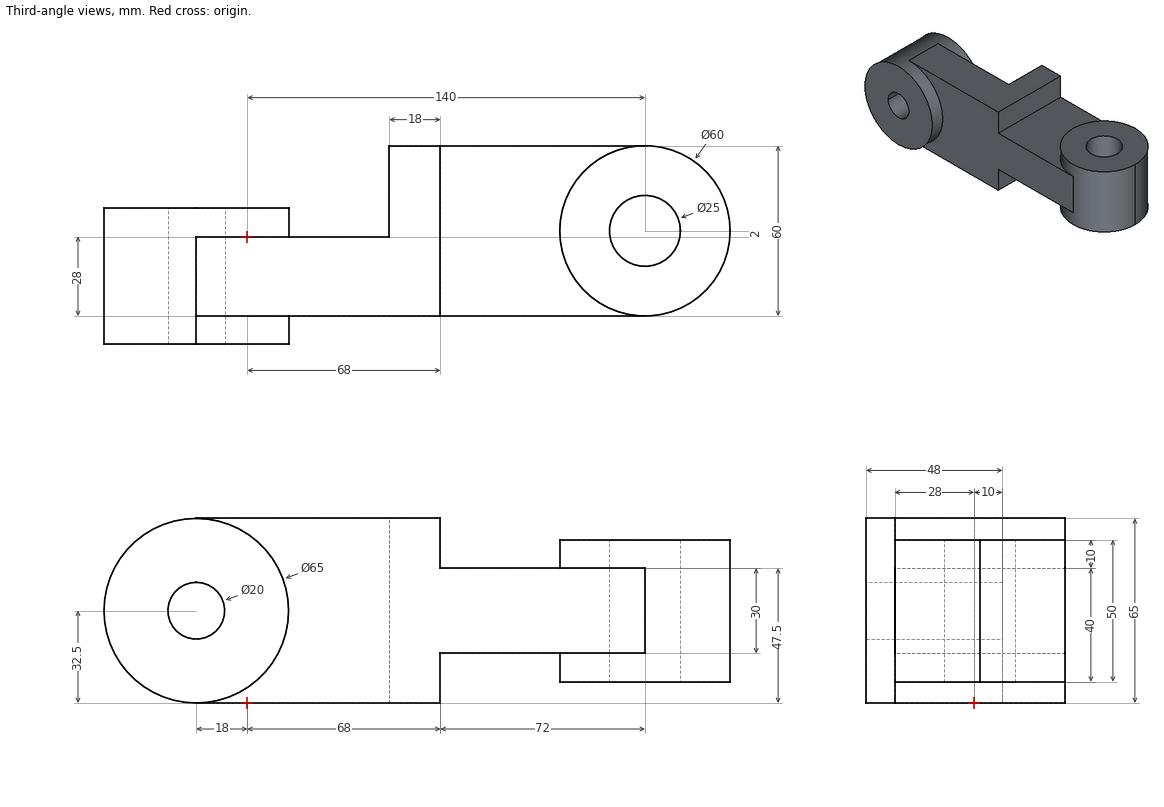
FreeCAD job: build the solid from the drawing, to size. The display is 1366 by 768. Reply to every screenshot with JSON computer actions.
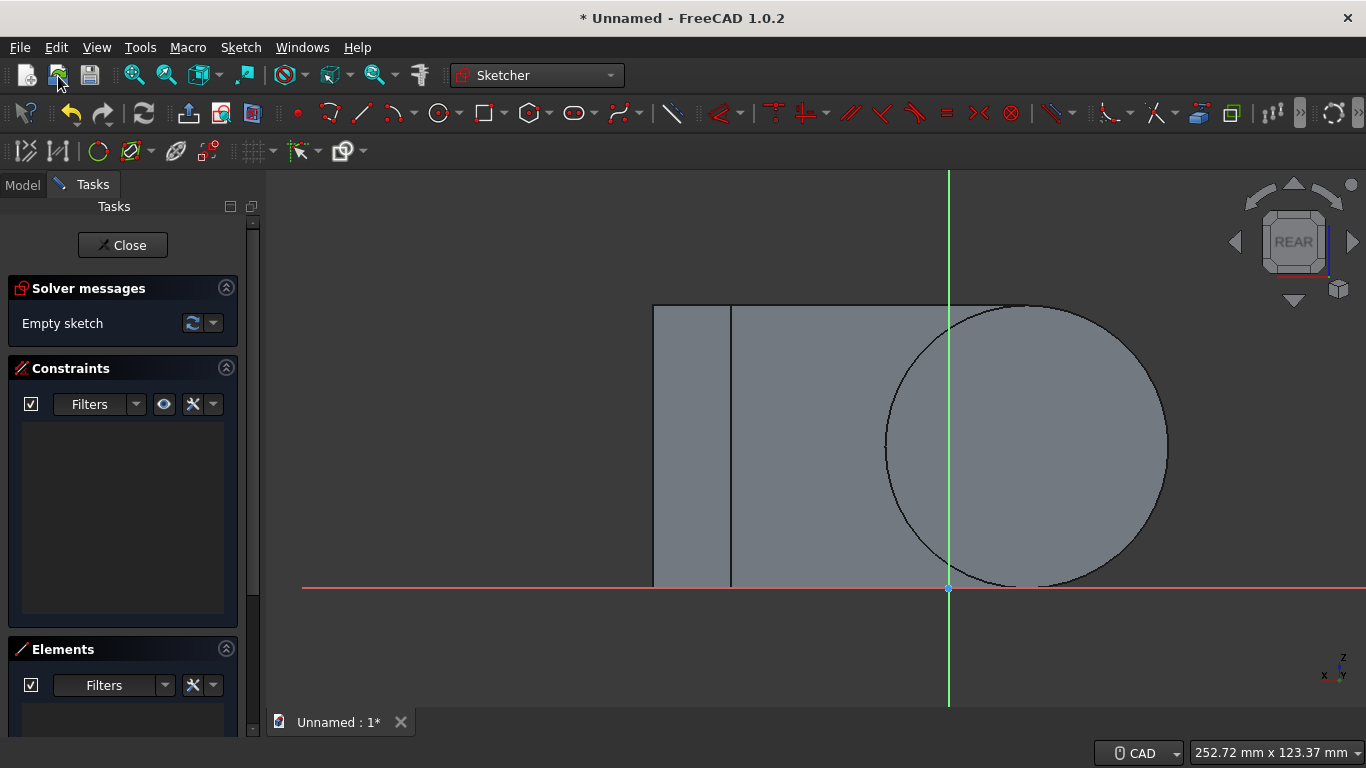
{"action": "scroll", "coordinate": [1201, 565], "scroll_direction": "up", "scroll_amount": 3}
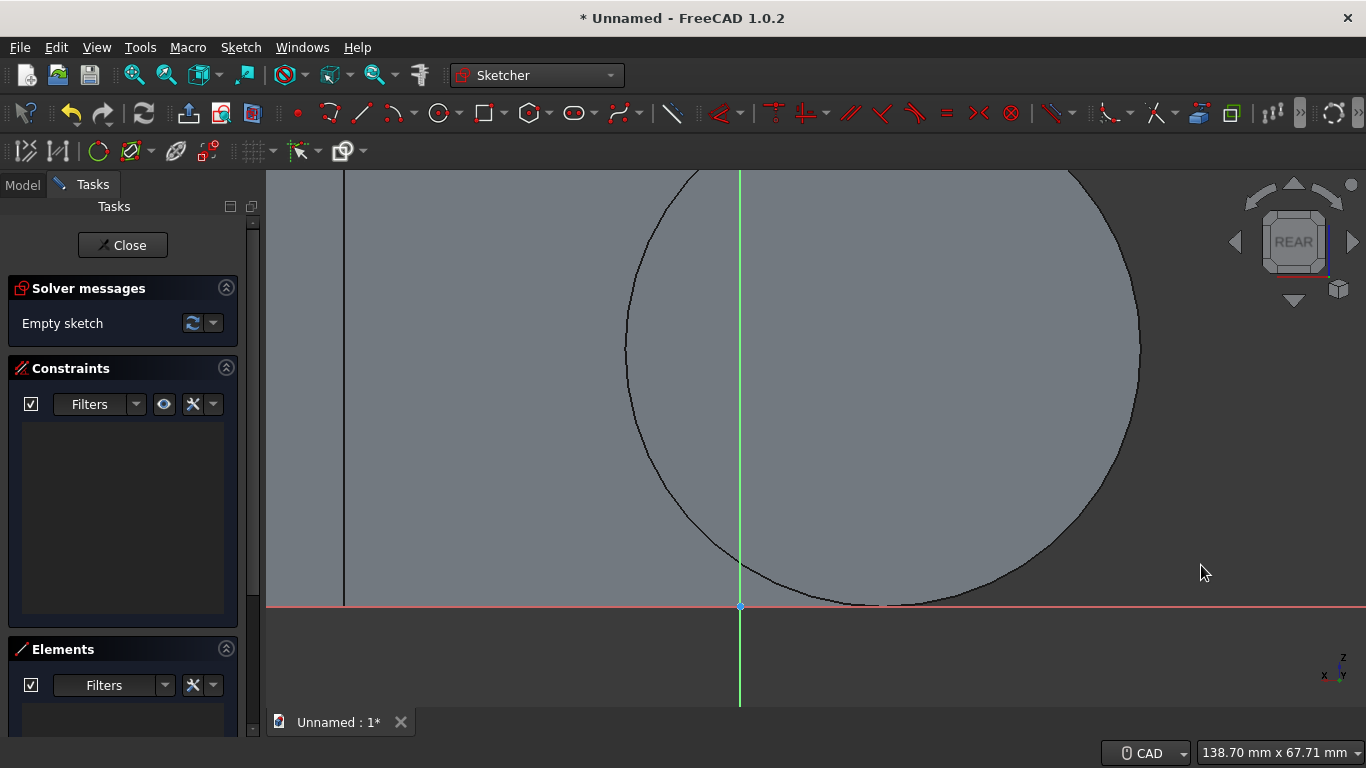
{"action": "key", "text": "g c"}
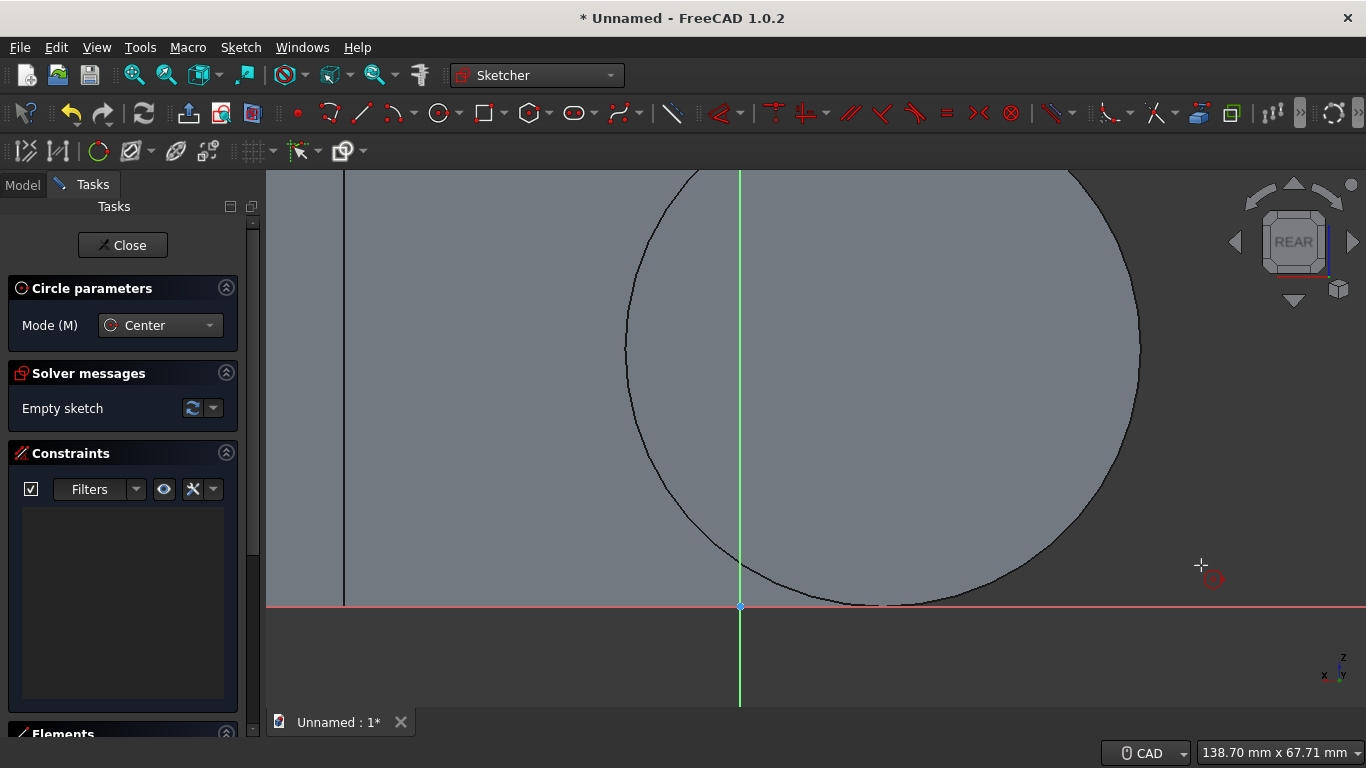
{"action": "left_click", "coordinate": [883, 349]}
{"action": "left_click", "coordinate": [939, 293]}
{"action": "key", "text": "Escape"}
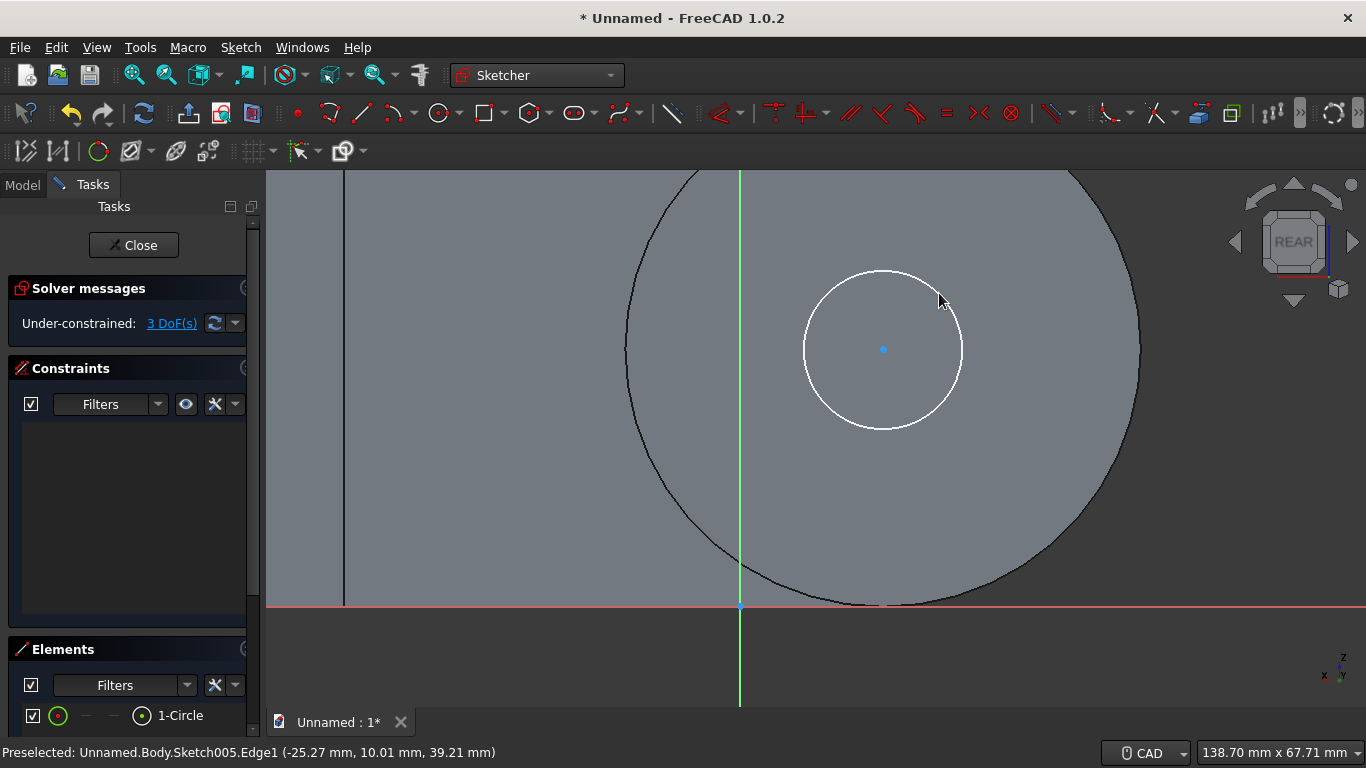
{"action": "key", "text": "d"}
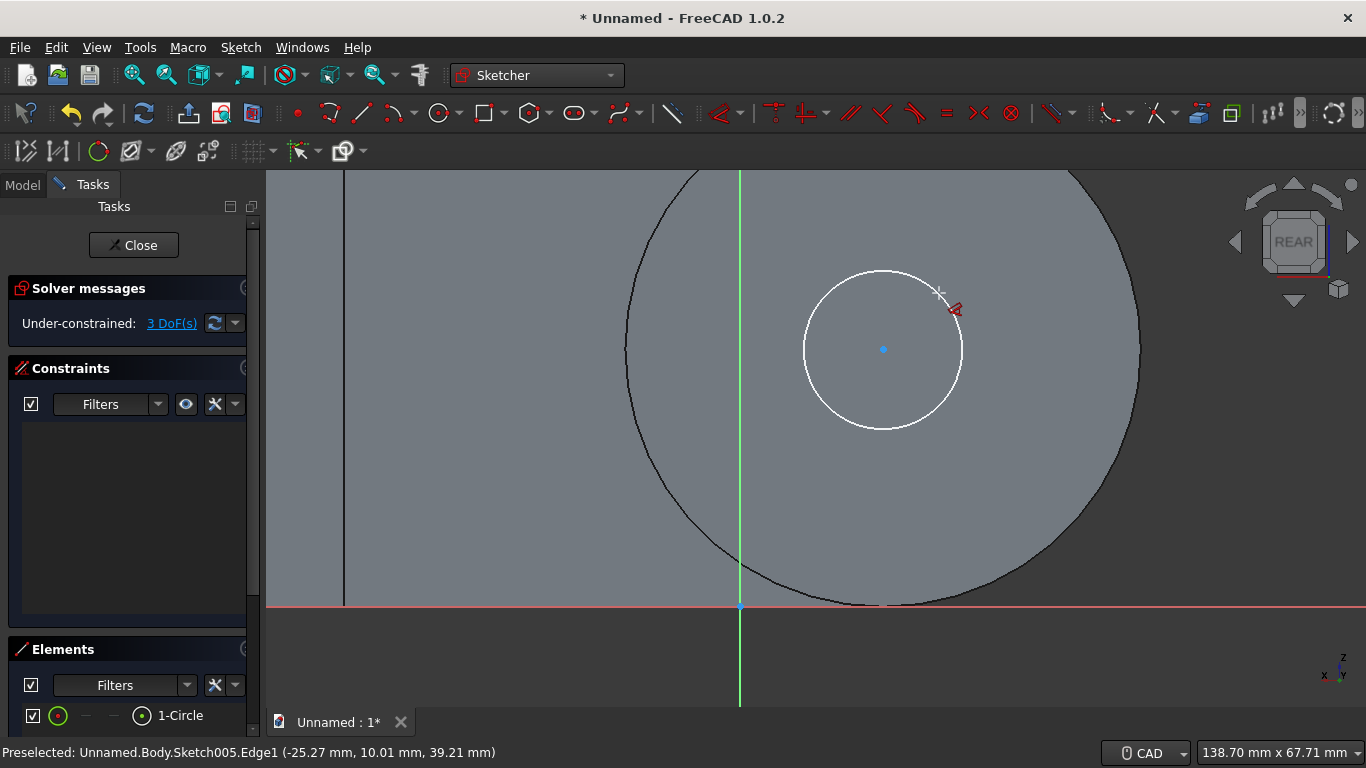
{"action": "left_click", "coordinate": [939, 294]}
{"action": "left_click", "coordinate": [962, 271]}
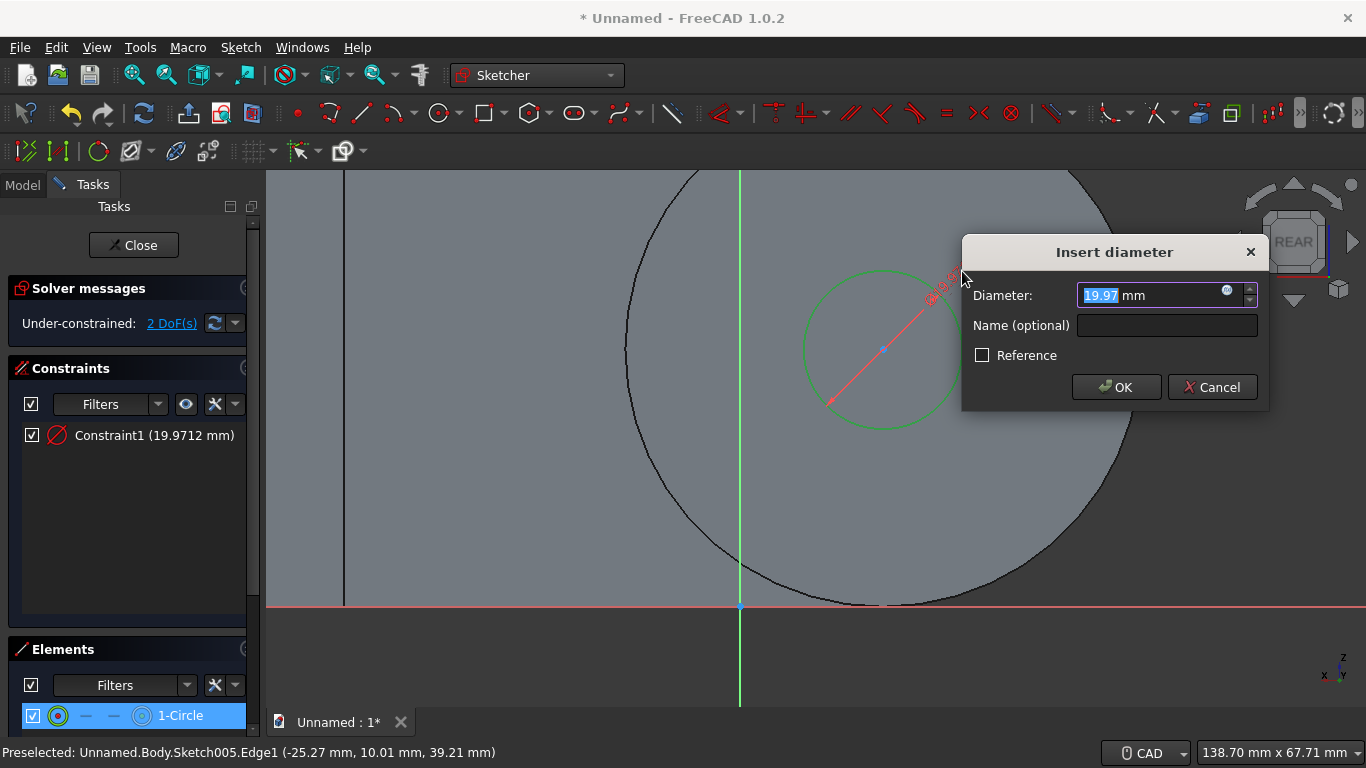
{"action": "type", "text": "20"}
{"action": "key", "text": "Return"}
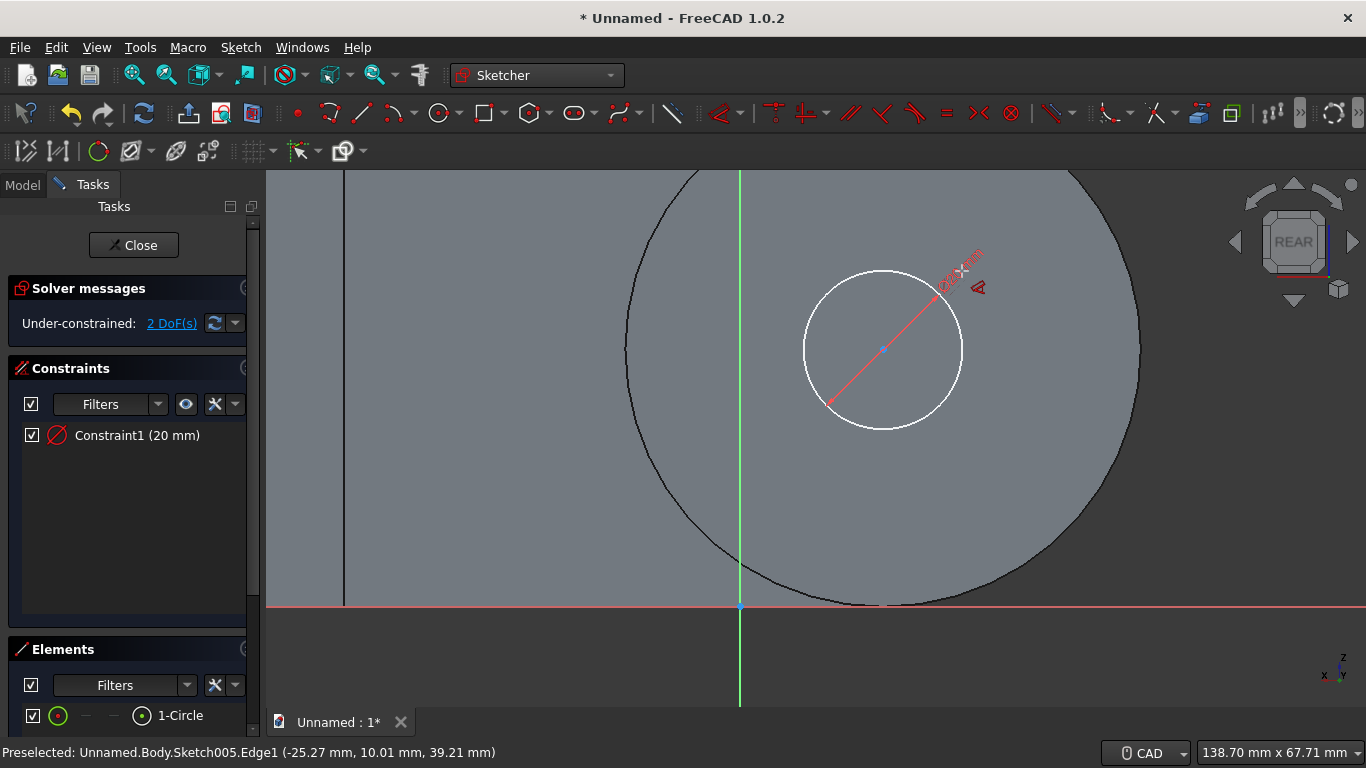
{"action": "left_click", "coordinate": [883, 350]}
{"action": "left_click", "coordinate": [812, 641]}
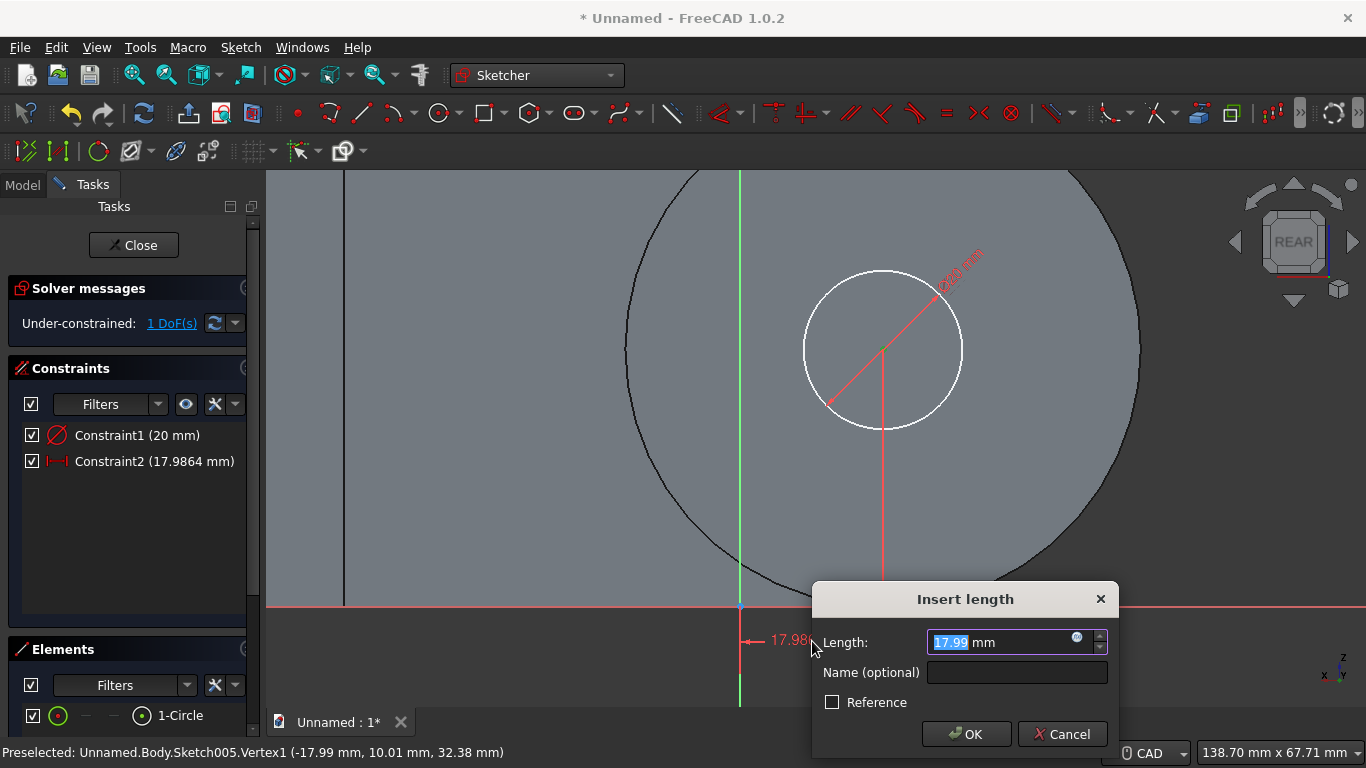
{"action": "type", "text": "18"}
{"action": "key", "text": "Return"}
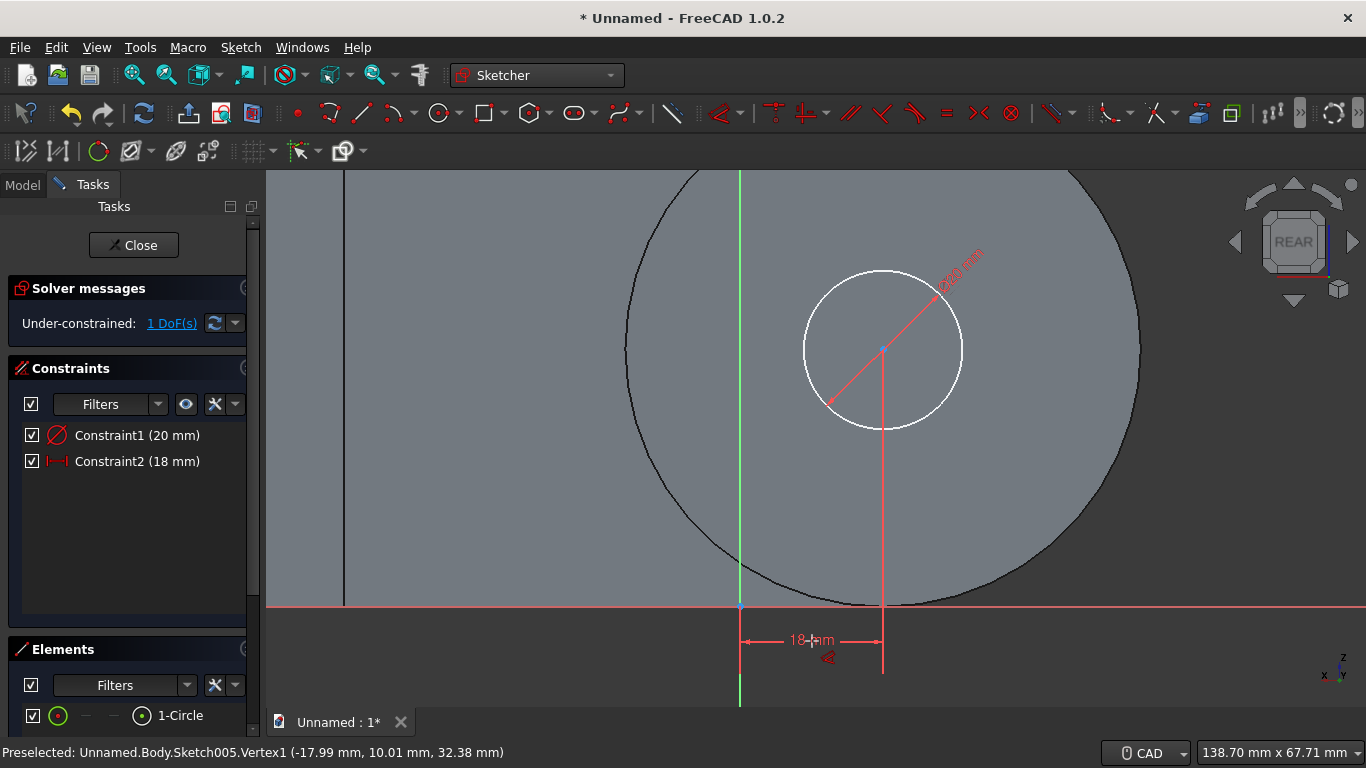
{"action": "left_click", "coordinate": [883, 350]}
{"action": "left_click", "coordinate": [706, 478]}